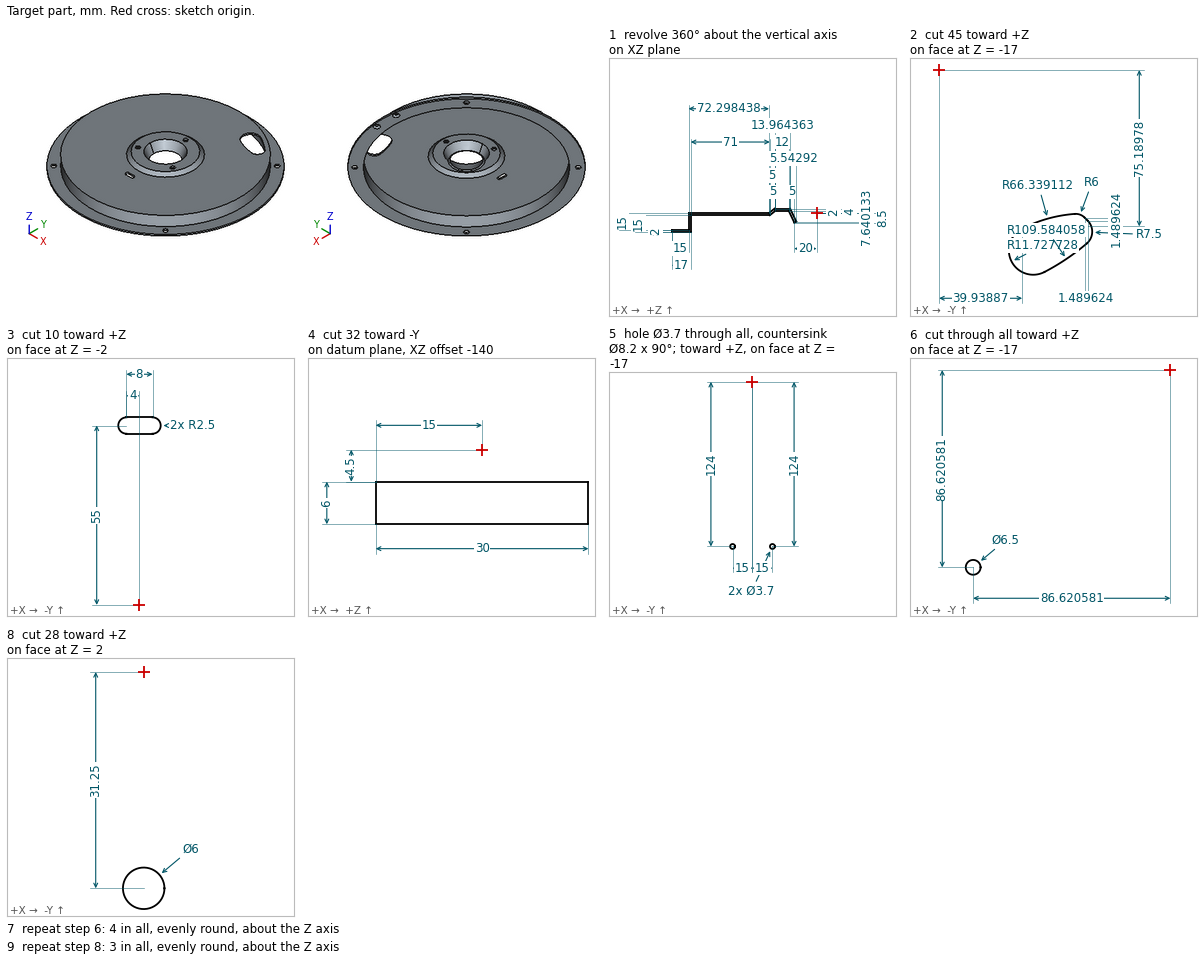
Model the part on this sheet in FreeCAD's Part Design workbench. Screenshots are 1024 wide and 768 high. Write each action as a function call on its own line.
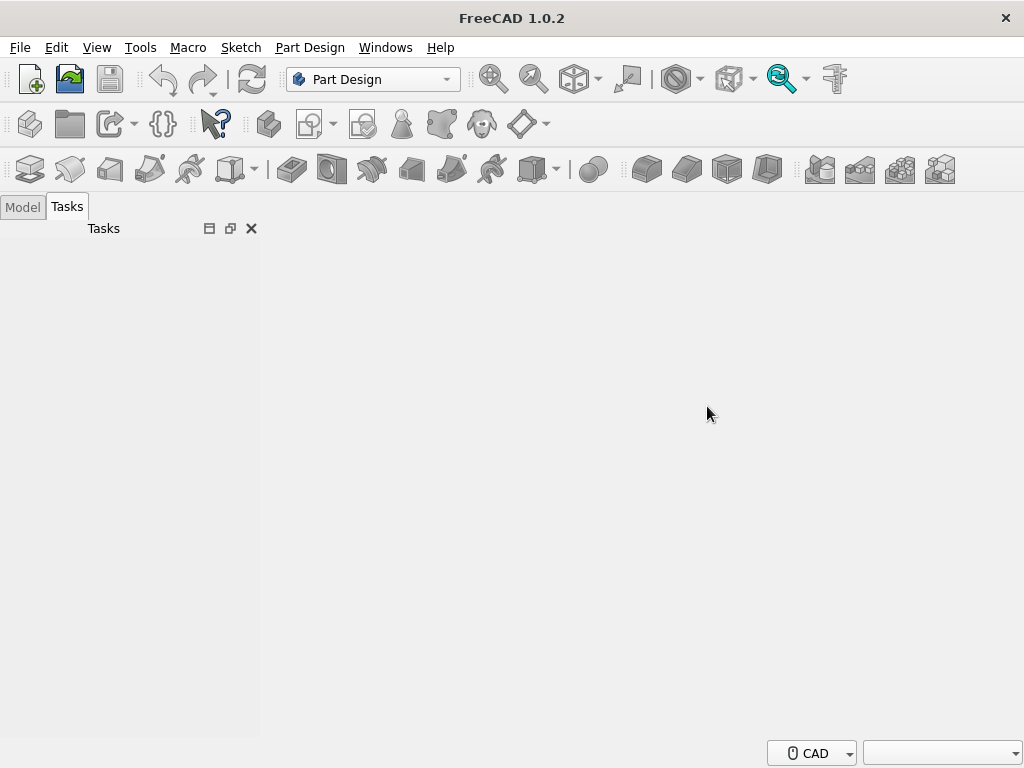
click(30, 80)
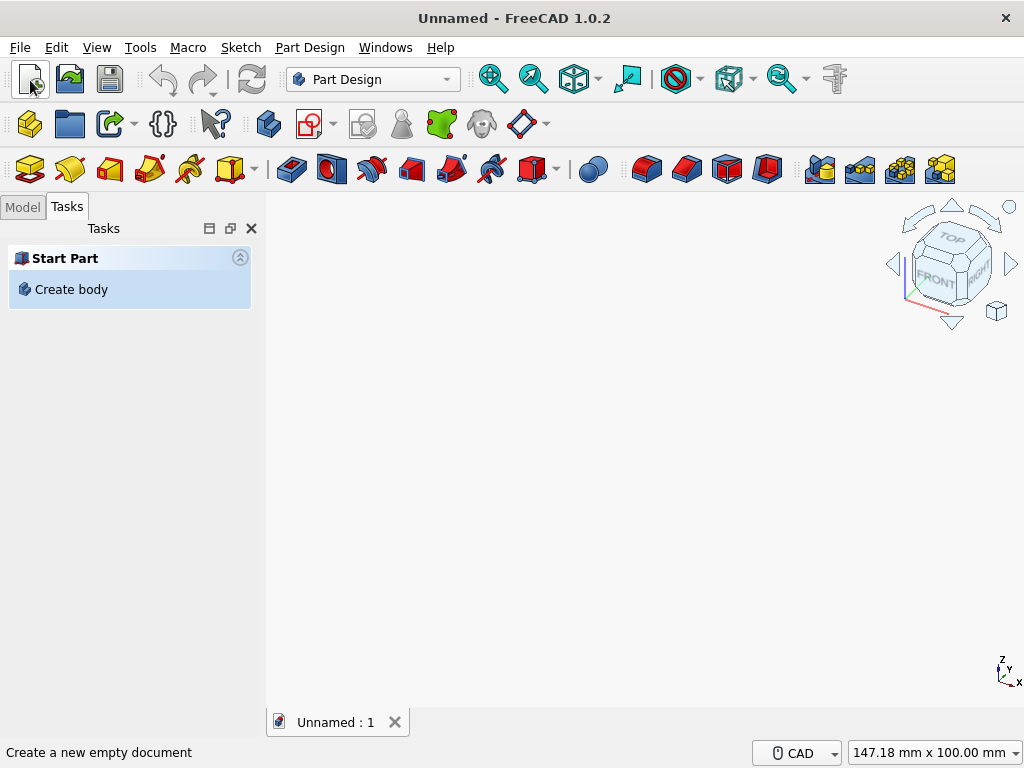
click(310, 124)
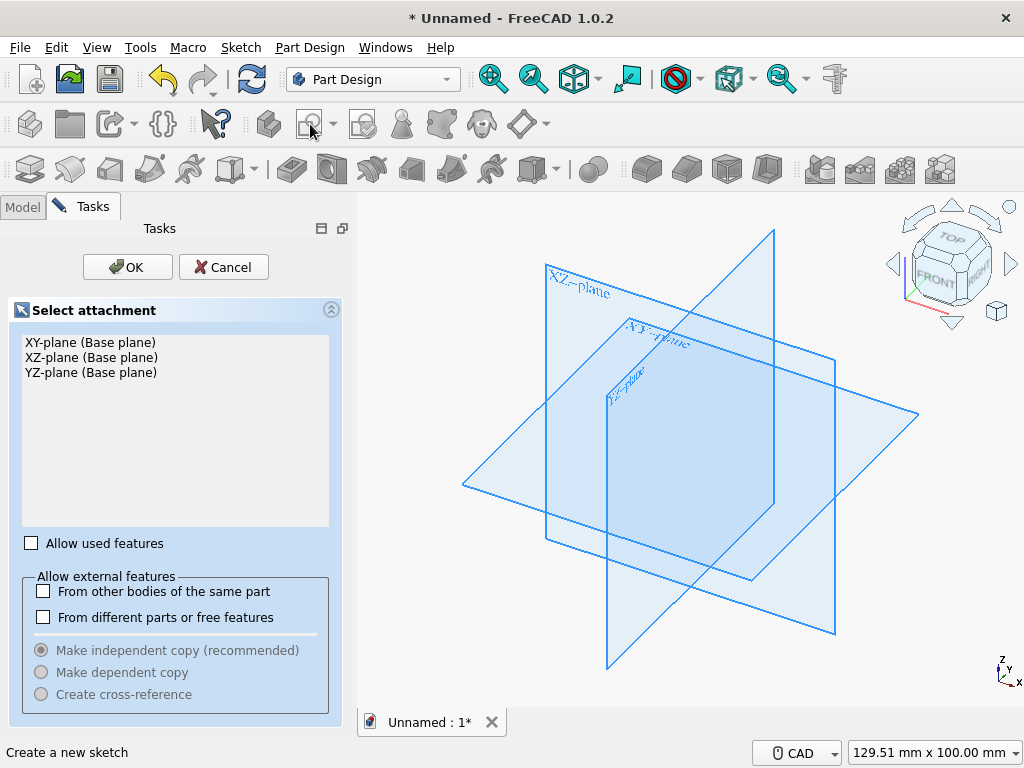
click(82, 358)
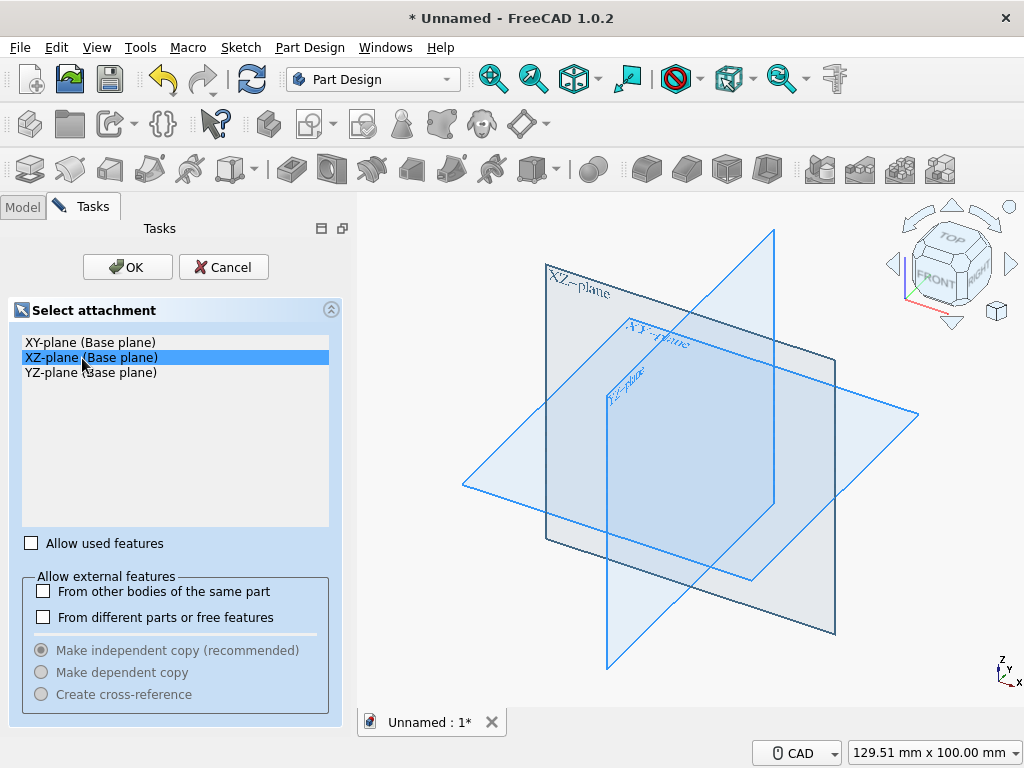
click(128, 267)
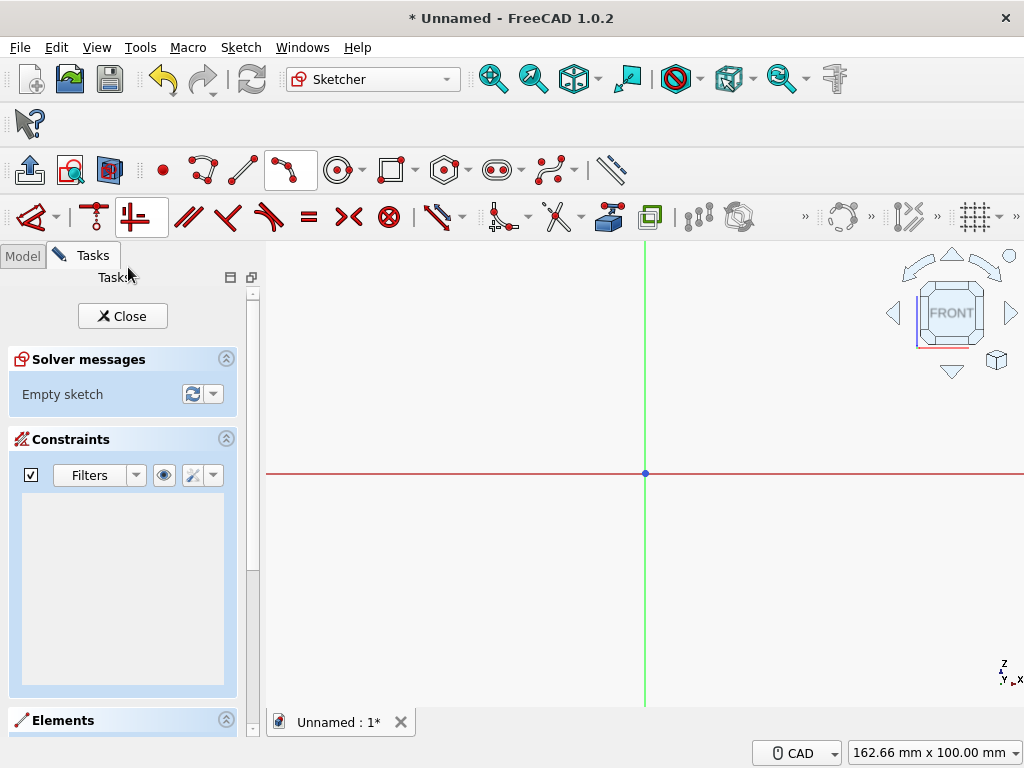
scroll(859, 437, down, 3)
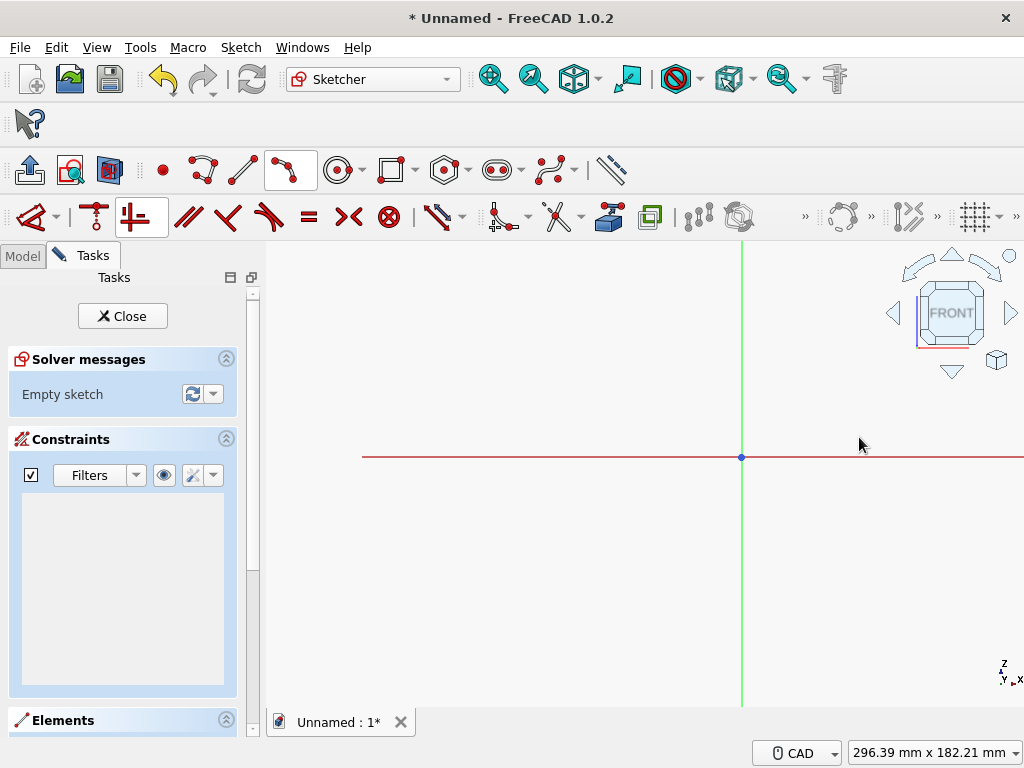
click(204, 170)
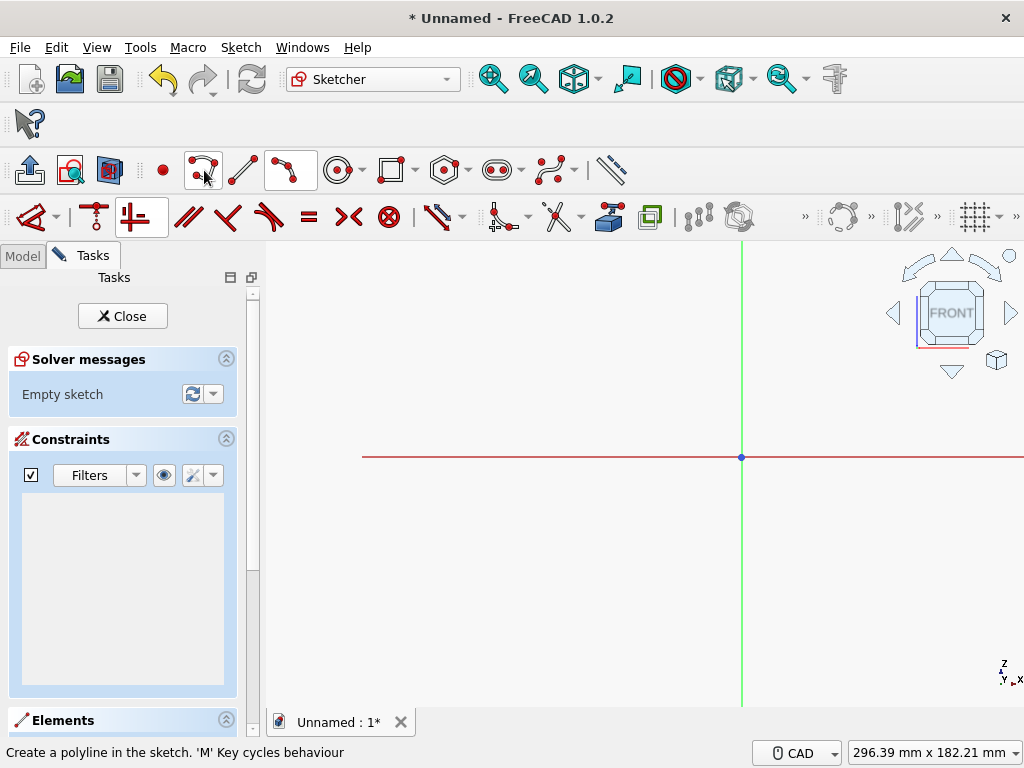
click(695, 477)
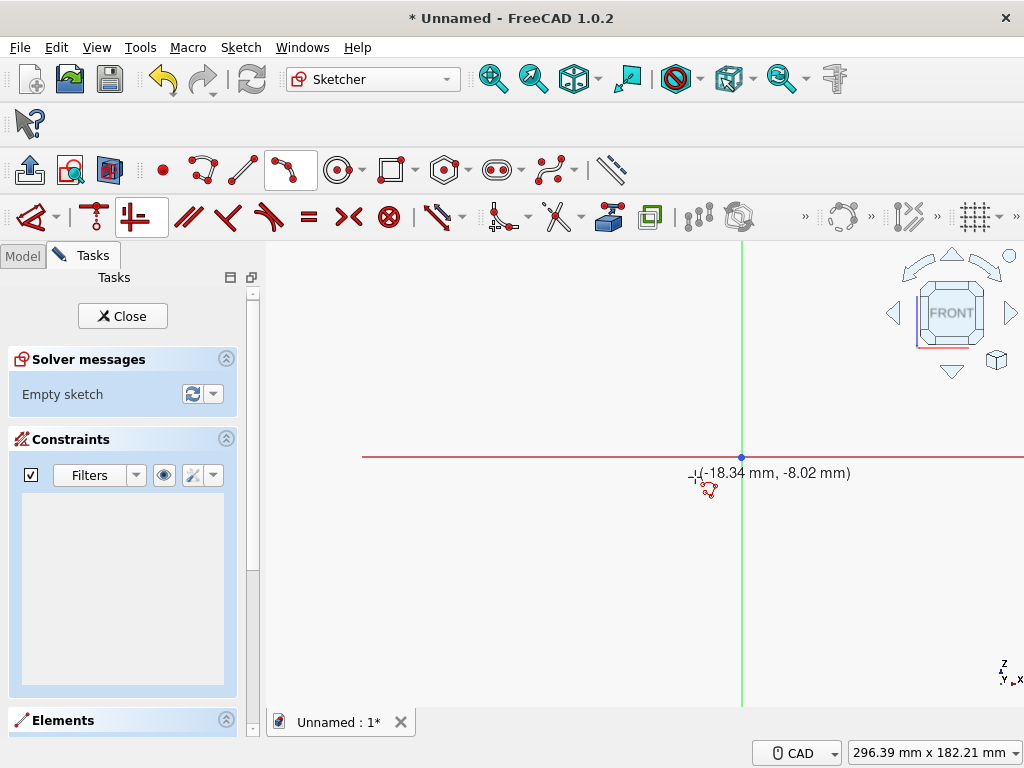
scroll(691, 479, up, 6)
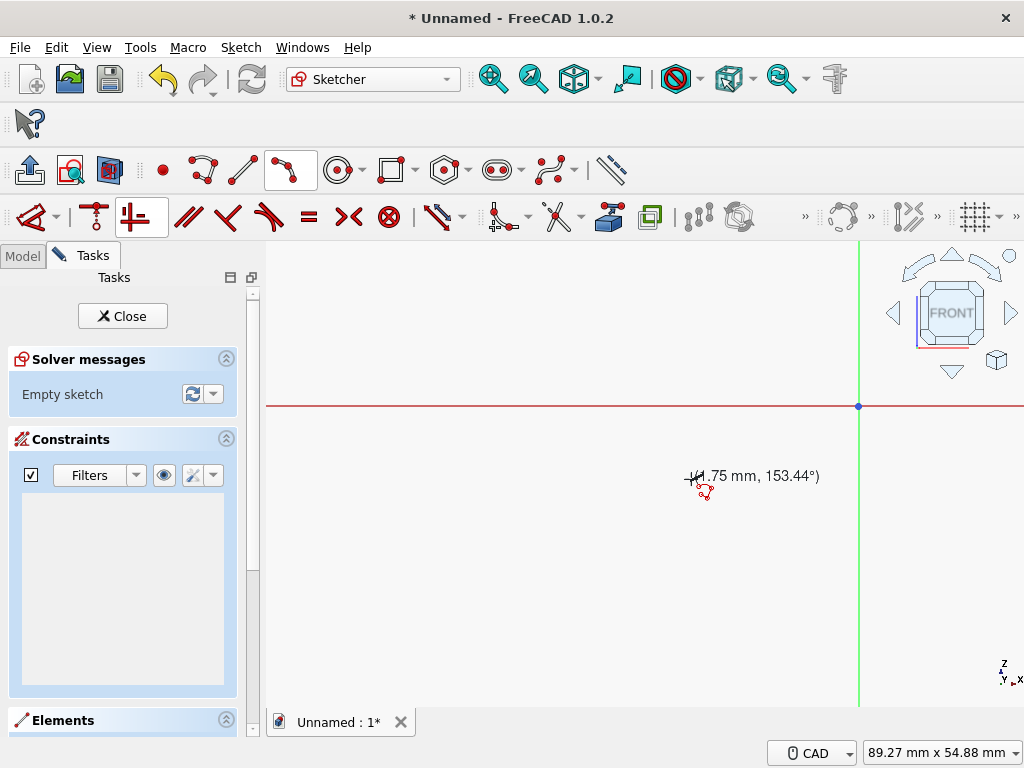
click(689, 479)
click(646, 389)
click(545, 389)
click(502, 423)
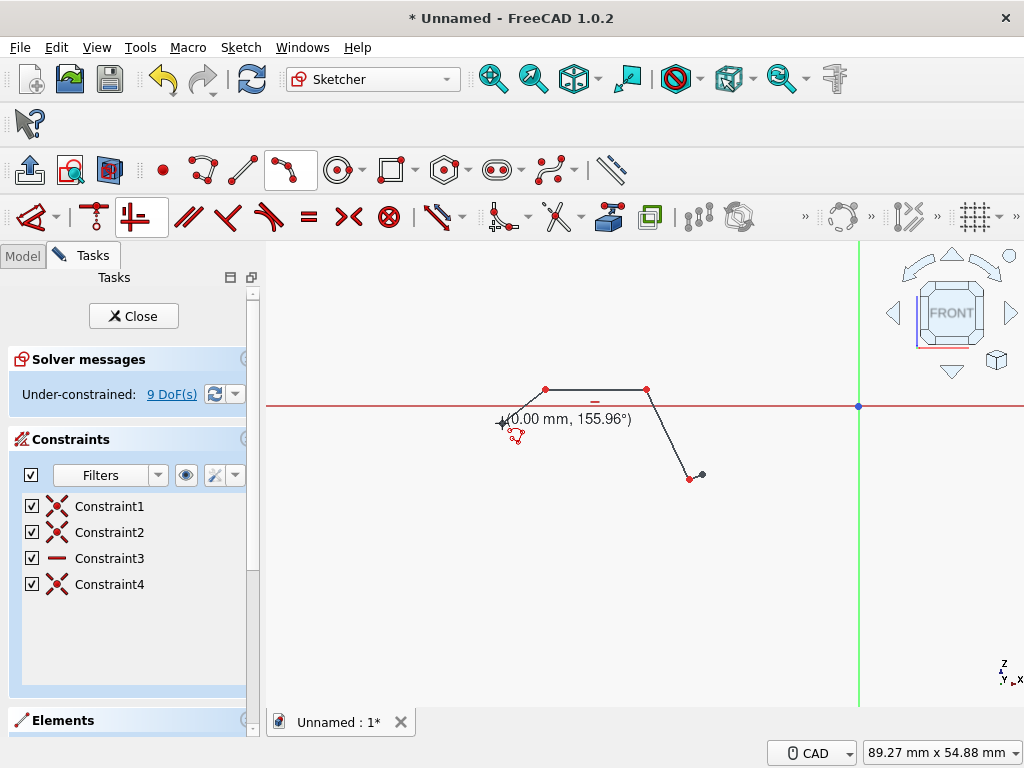
scroll(733, 481, down, 5)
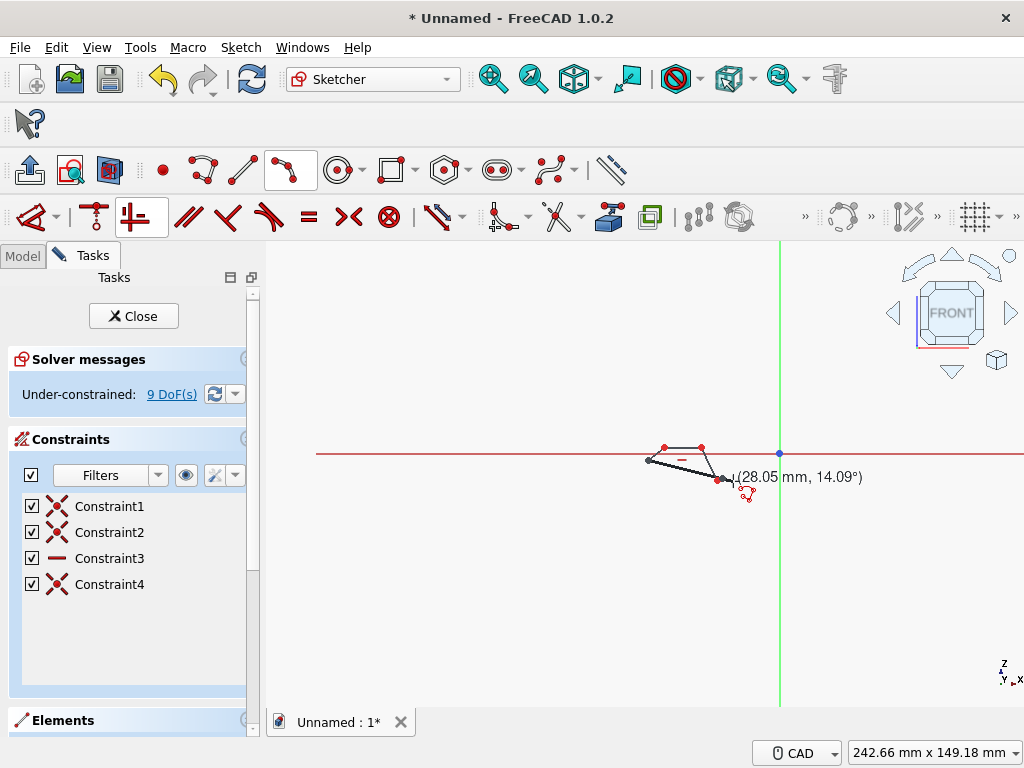
scroll(427, 460, up, 5)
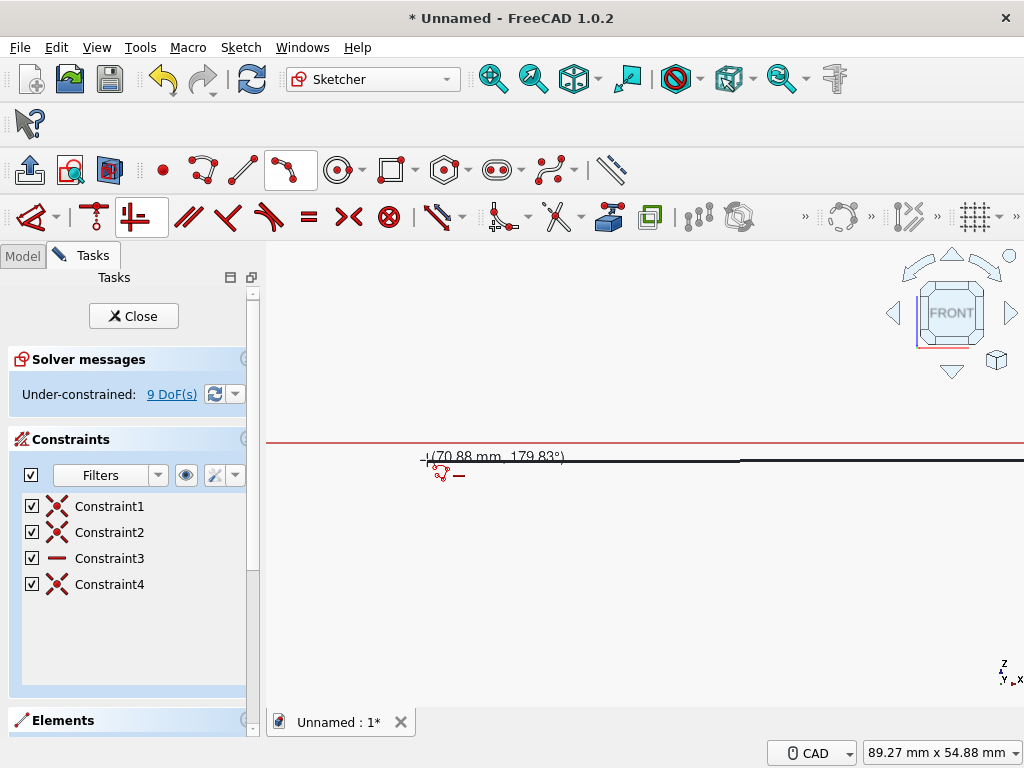
click(426, 459)
click(426, 587)